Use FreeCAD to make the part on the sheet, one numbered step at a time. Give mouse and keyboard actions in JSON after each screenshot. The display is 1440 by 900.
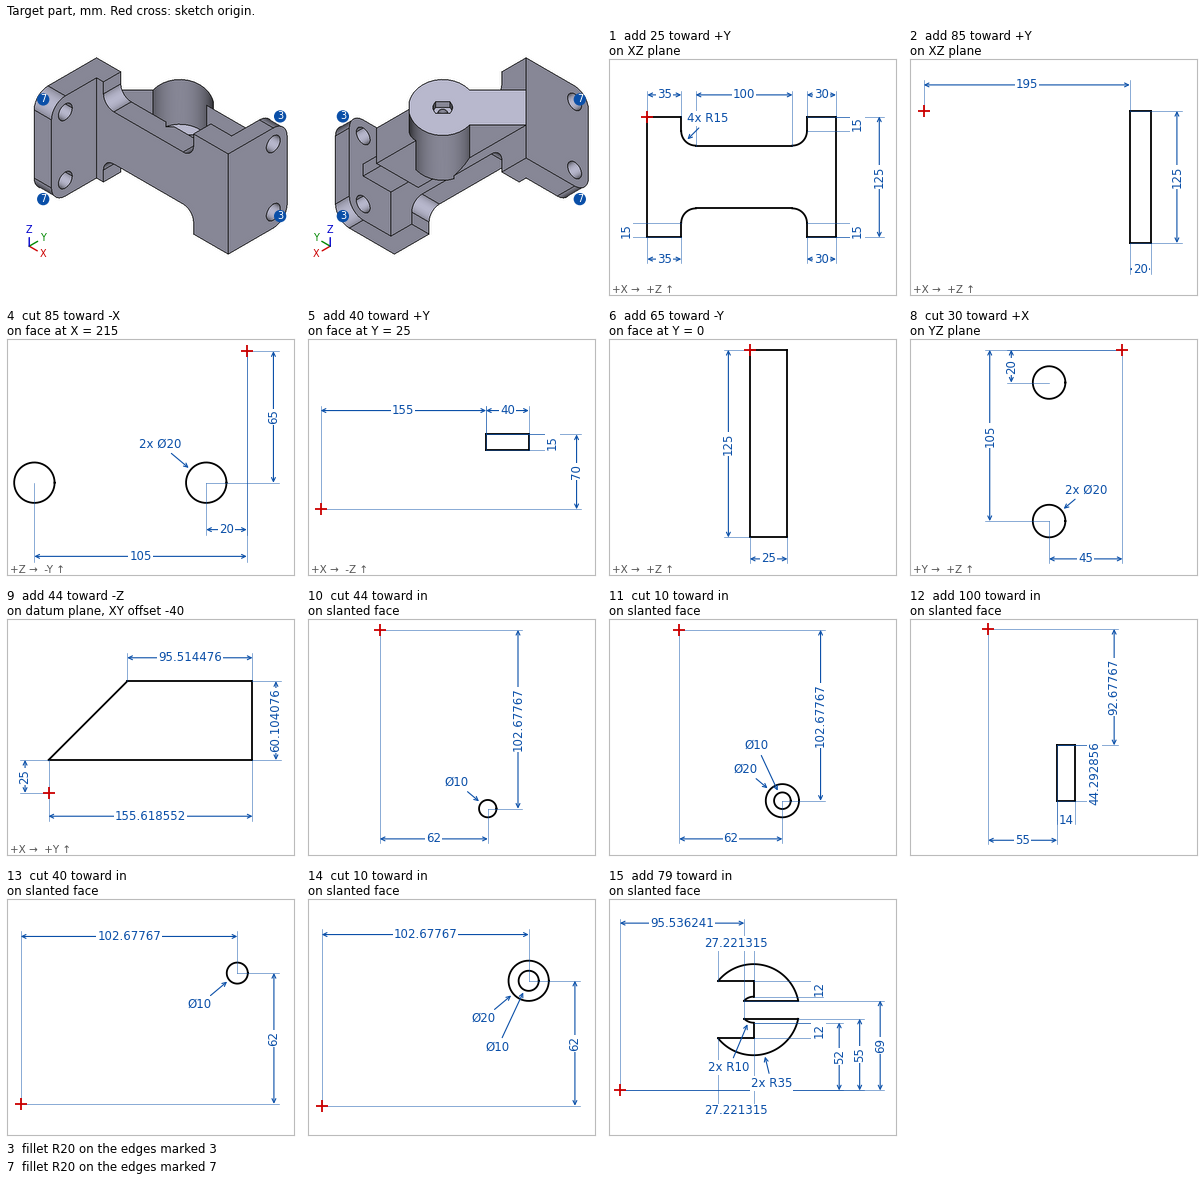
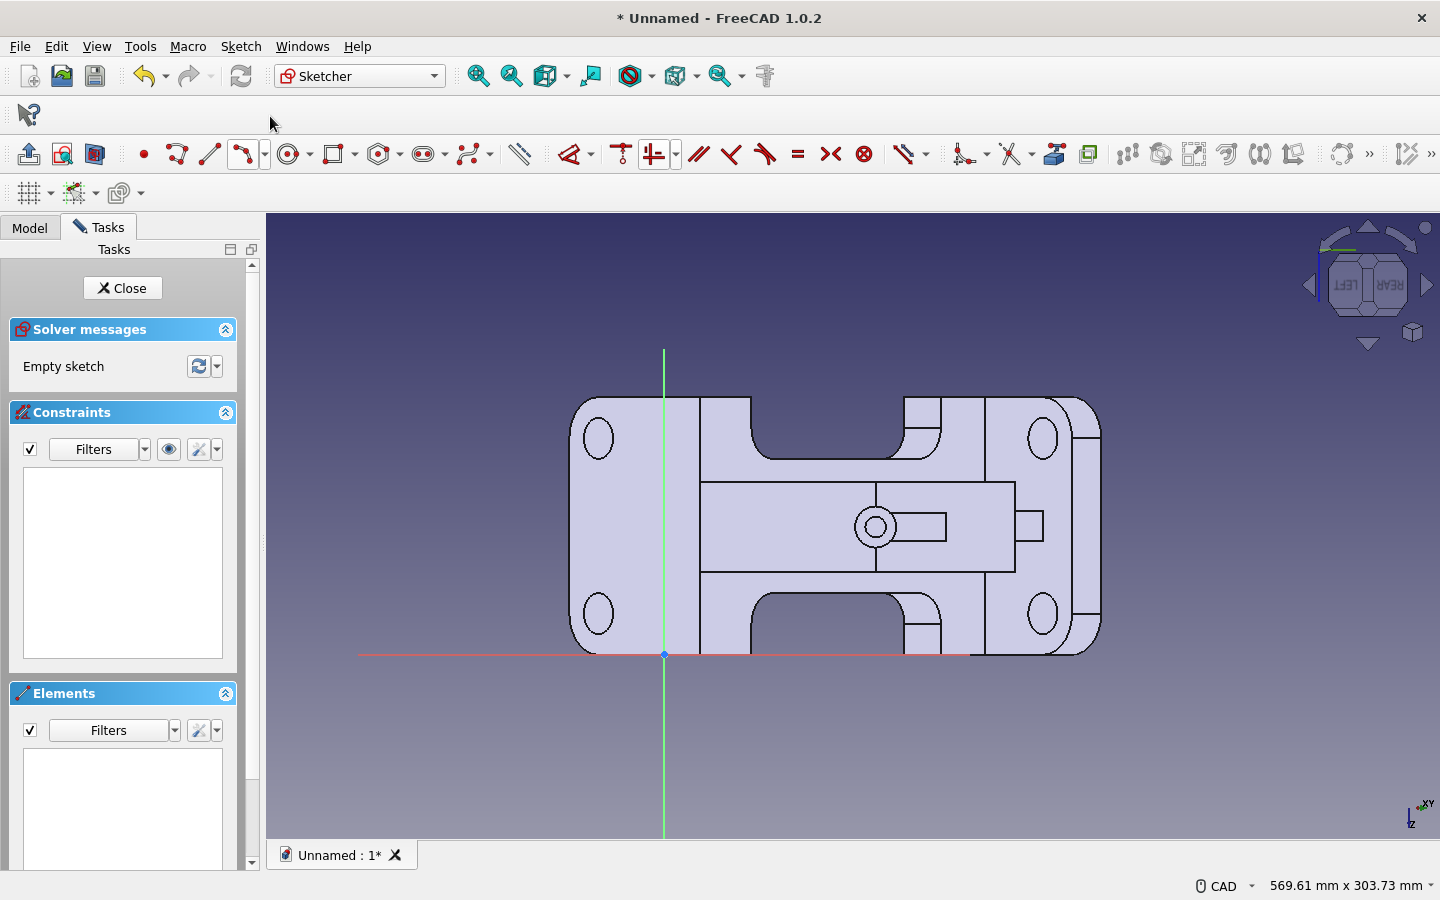
{"action": "scroll", "coordinate": [822, 580], "scroll_direction": "up", "scroll_amount": 4}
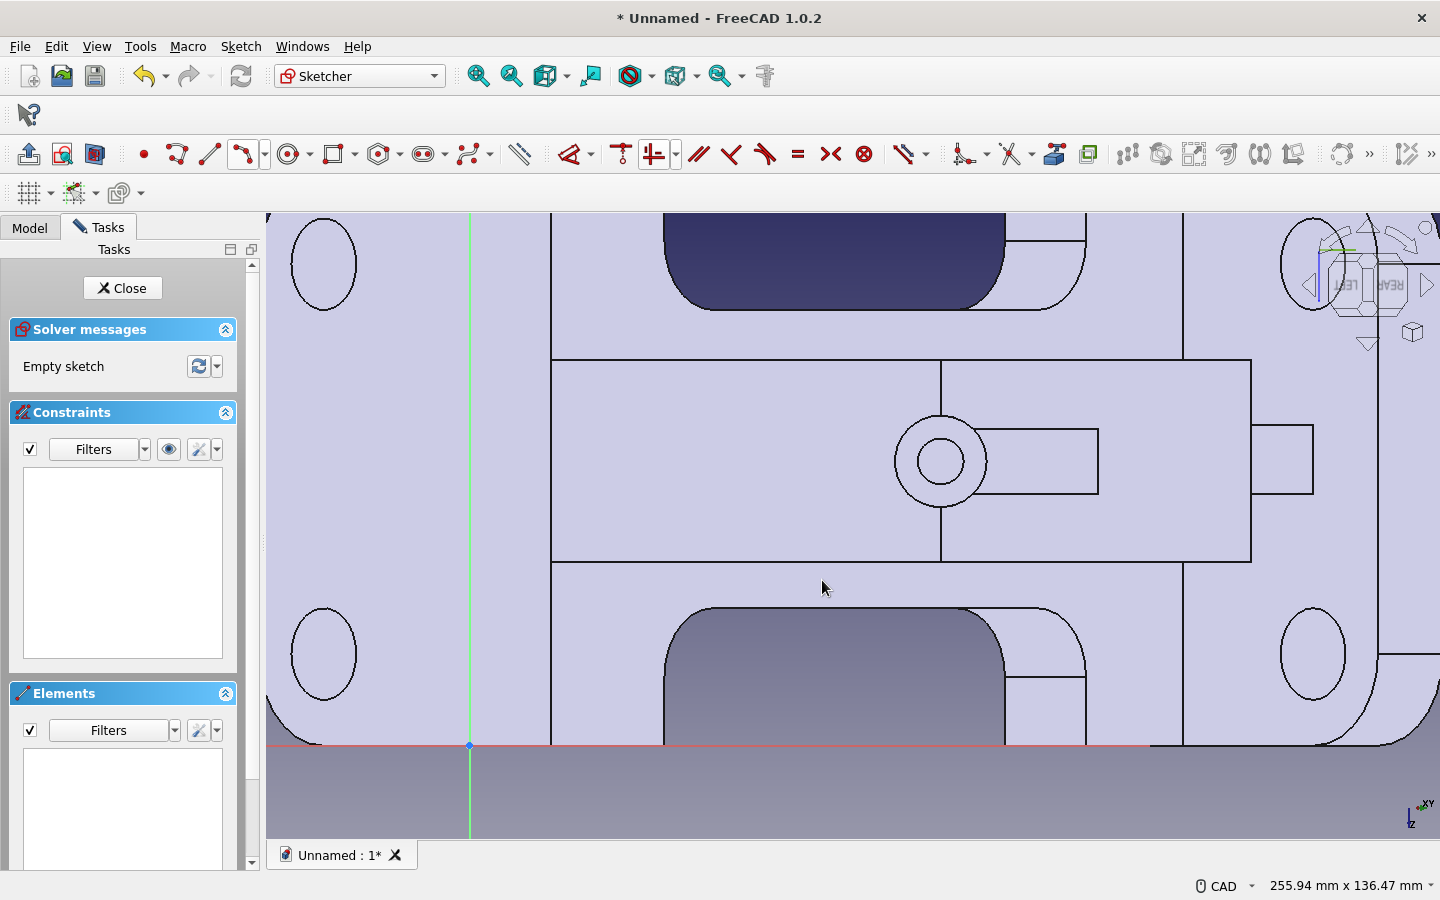
{"action": "left_click", "coordinate": [210, 154]}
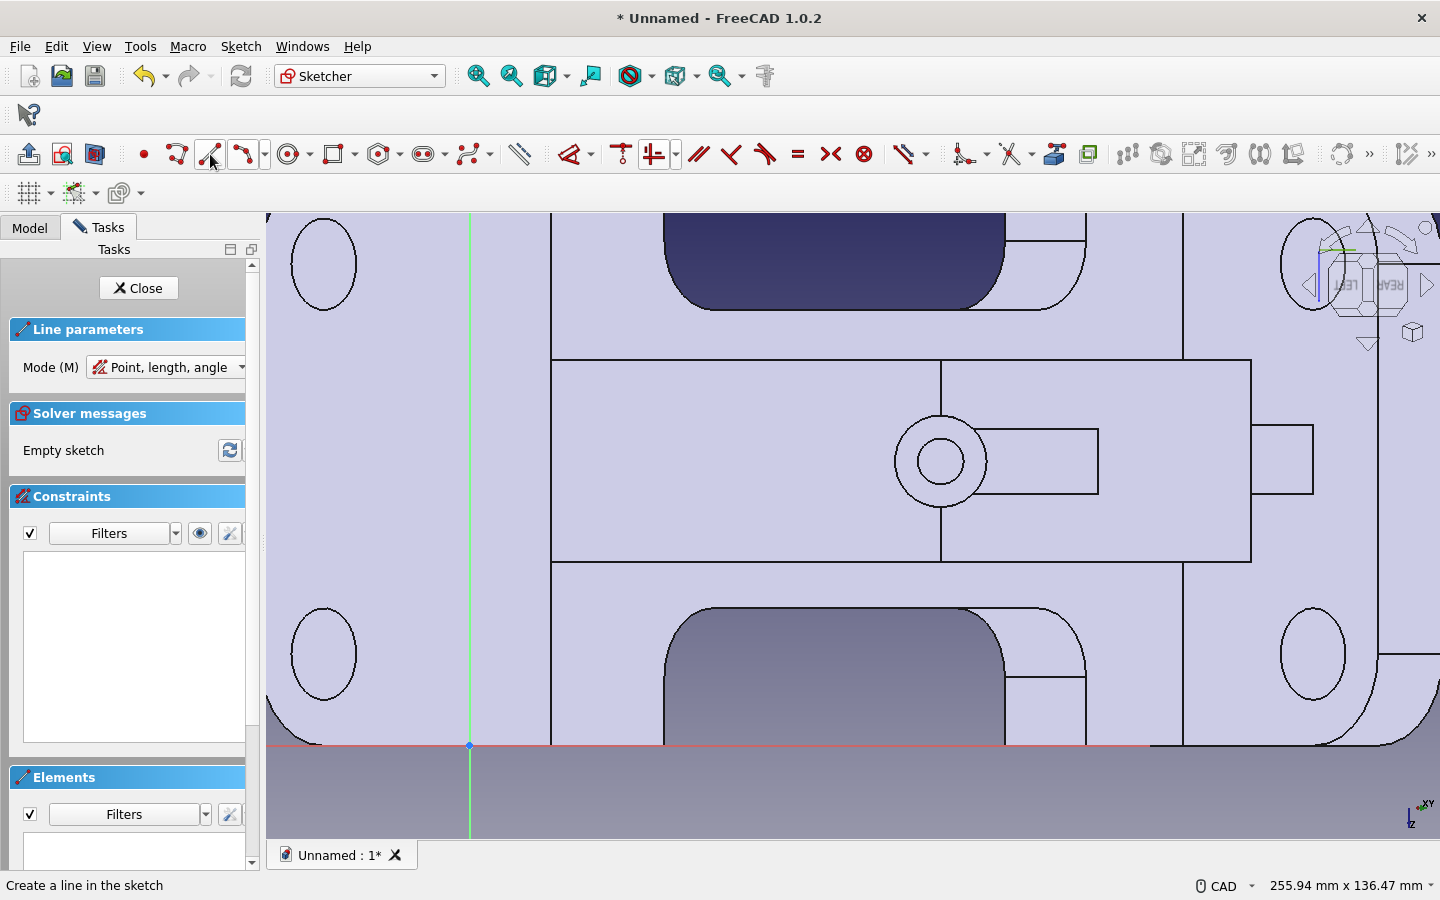
{"action": "left_click", "coordinate": [1098, 494]}
{"action": "left_click", "coordinate": [908, 494]}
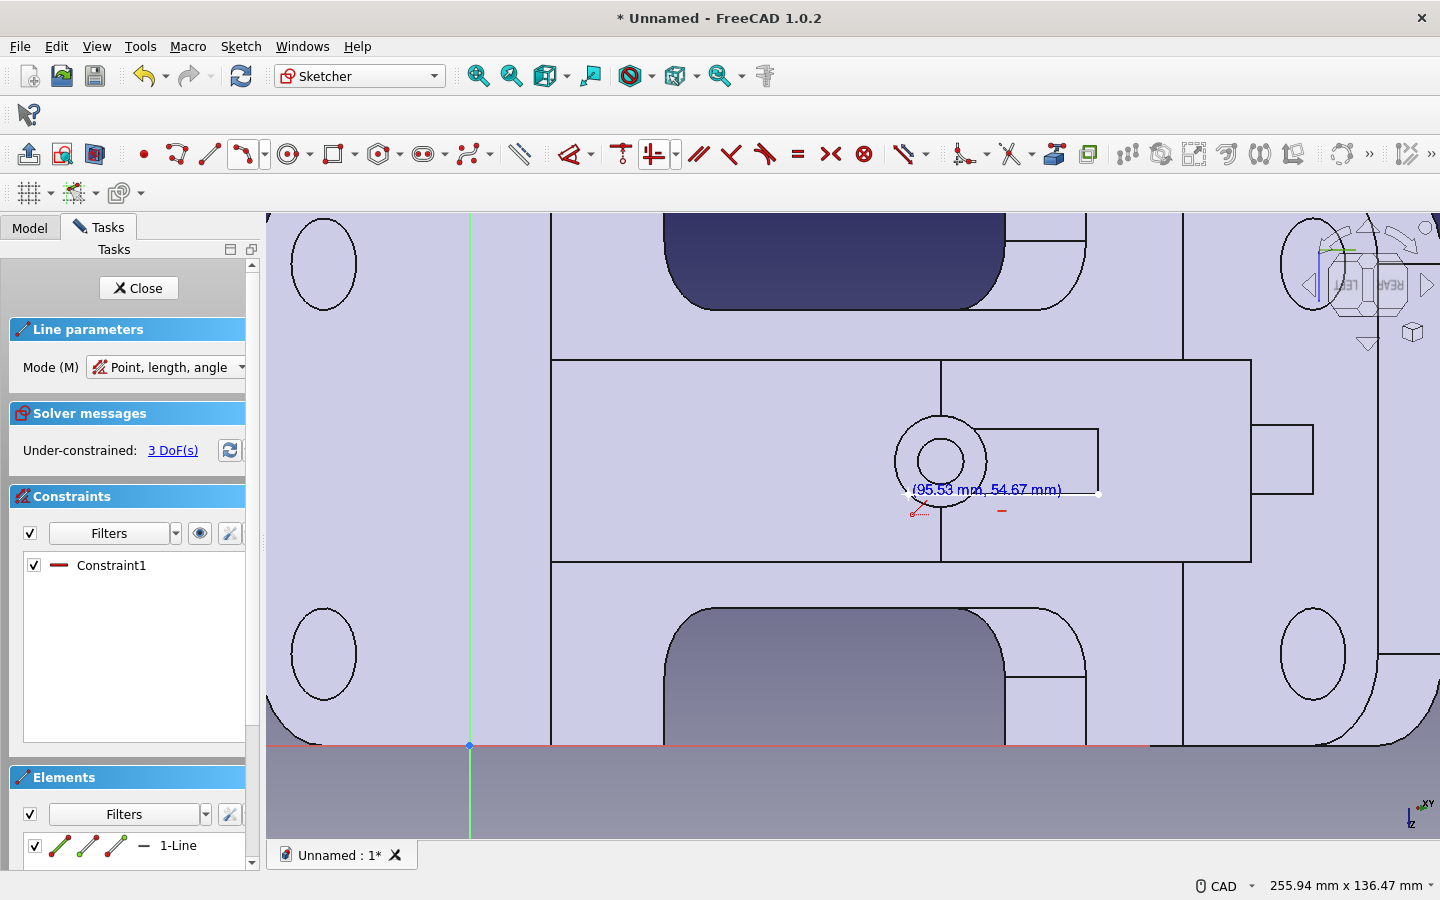
{"action": "left_click", "coordinate": [177, 154]}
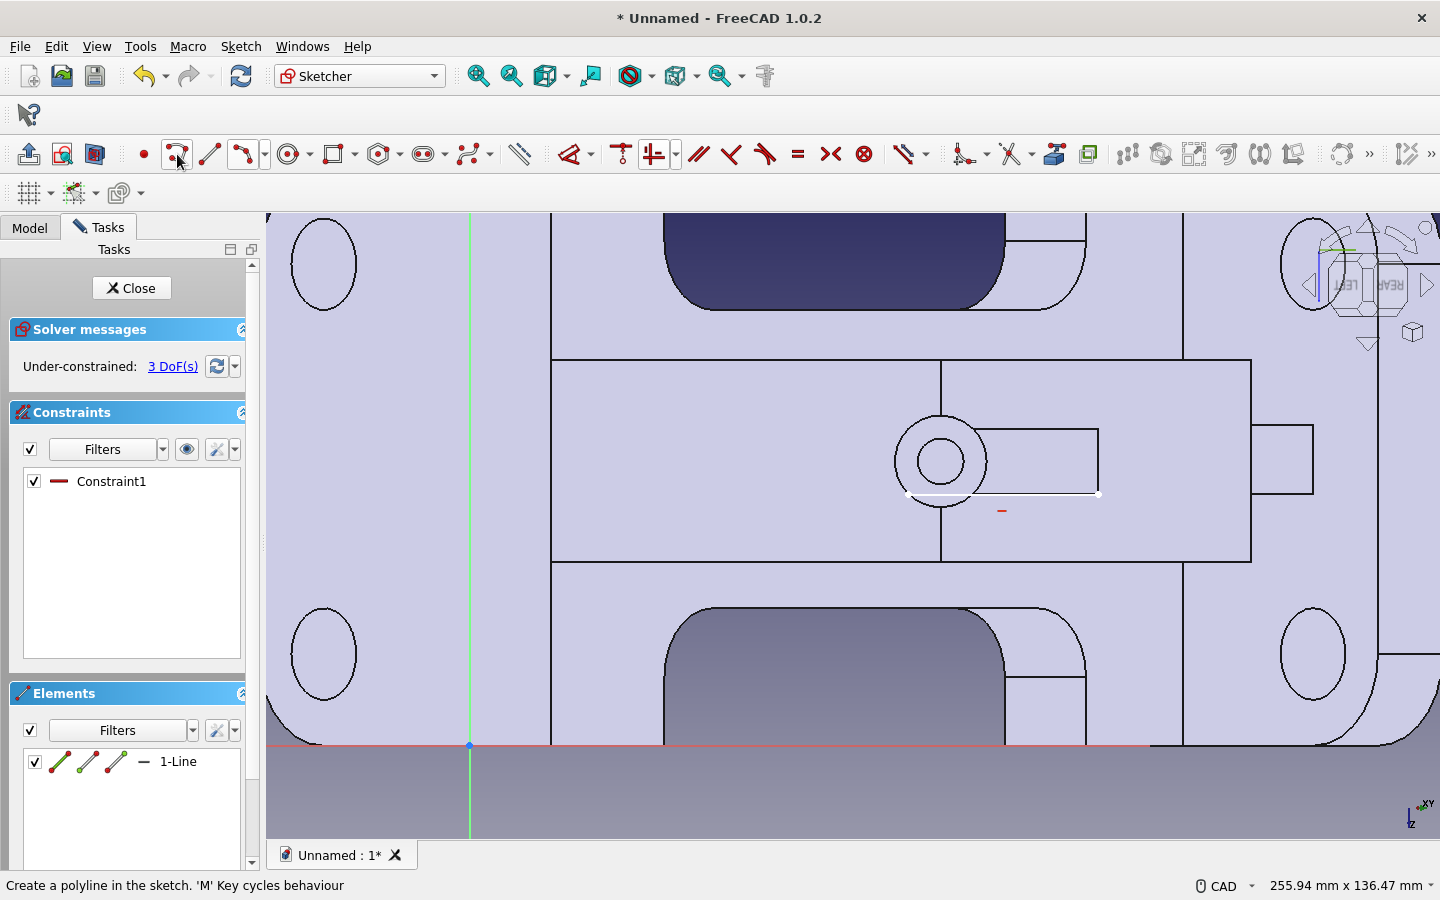
{"action": "left_click", "coordinate": [941, 507]}
{"action": "left_click", "coordinate": [941, 562]}
{"action": "left_click", "coordinate": [816, 562]}
{"action": "right_click", "coordinate": [816, 562]}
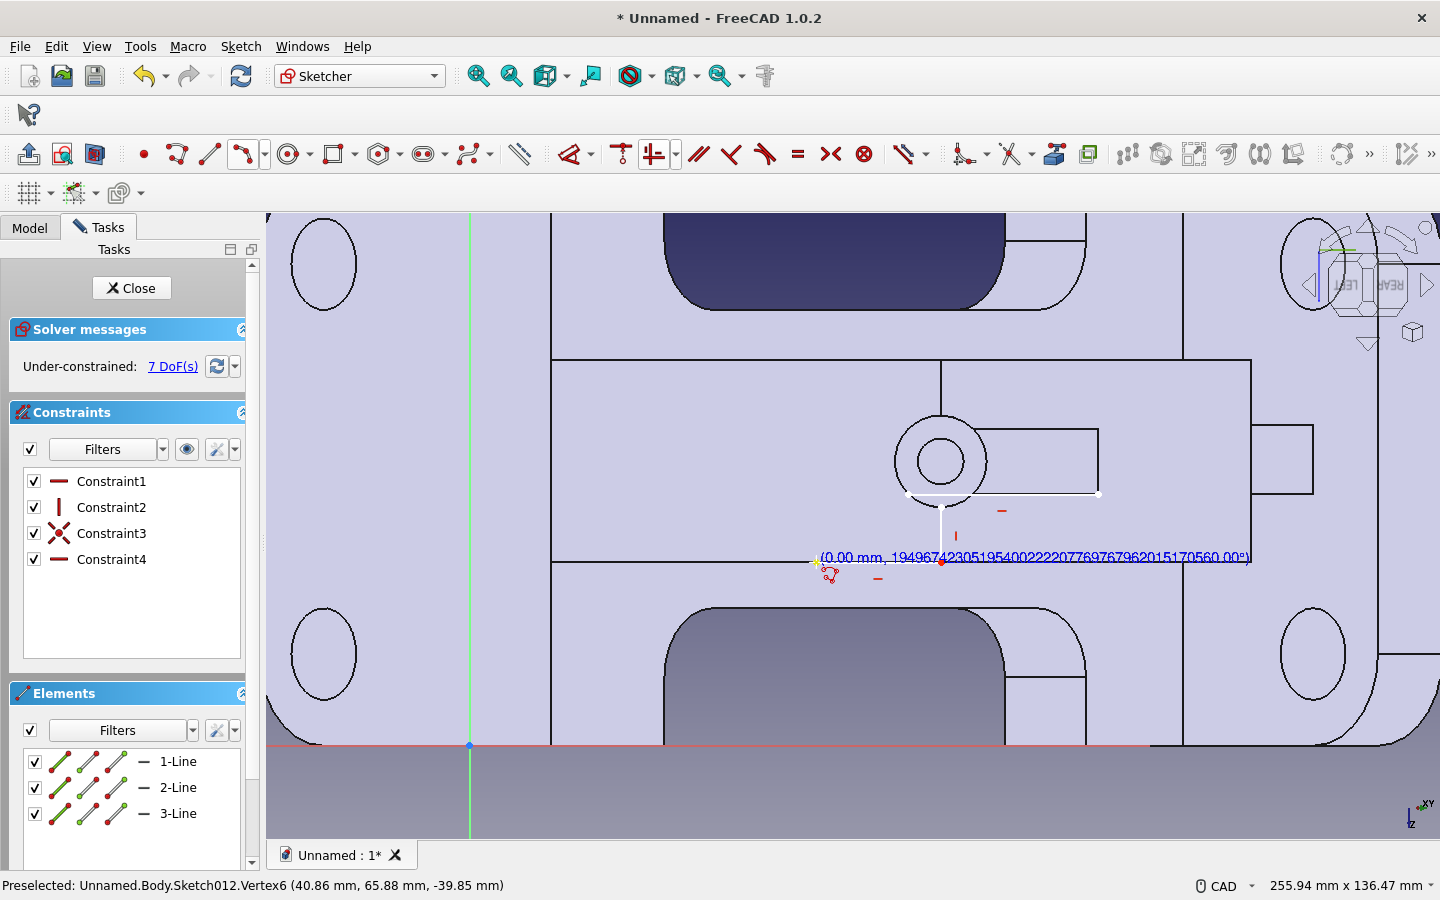
{"action": "left_click", "coordinate": [242, 154]}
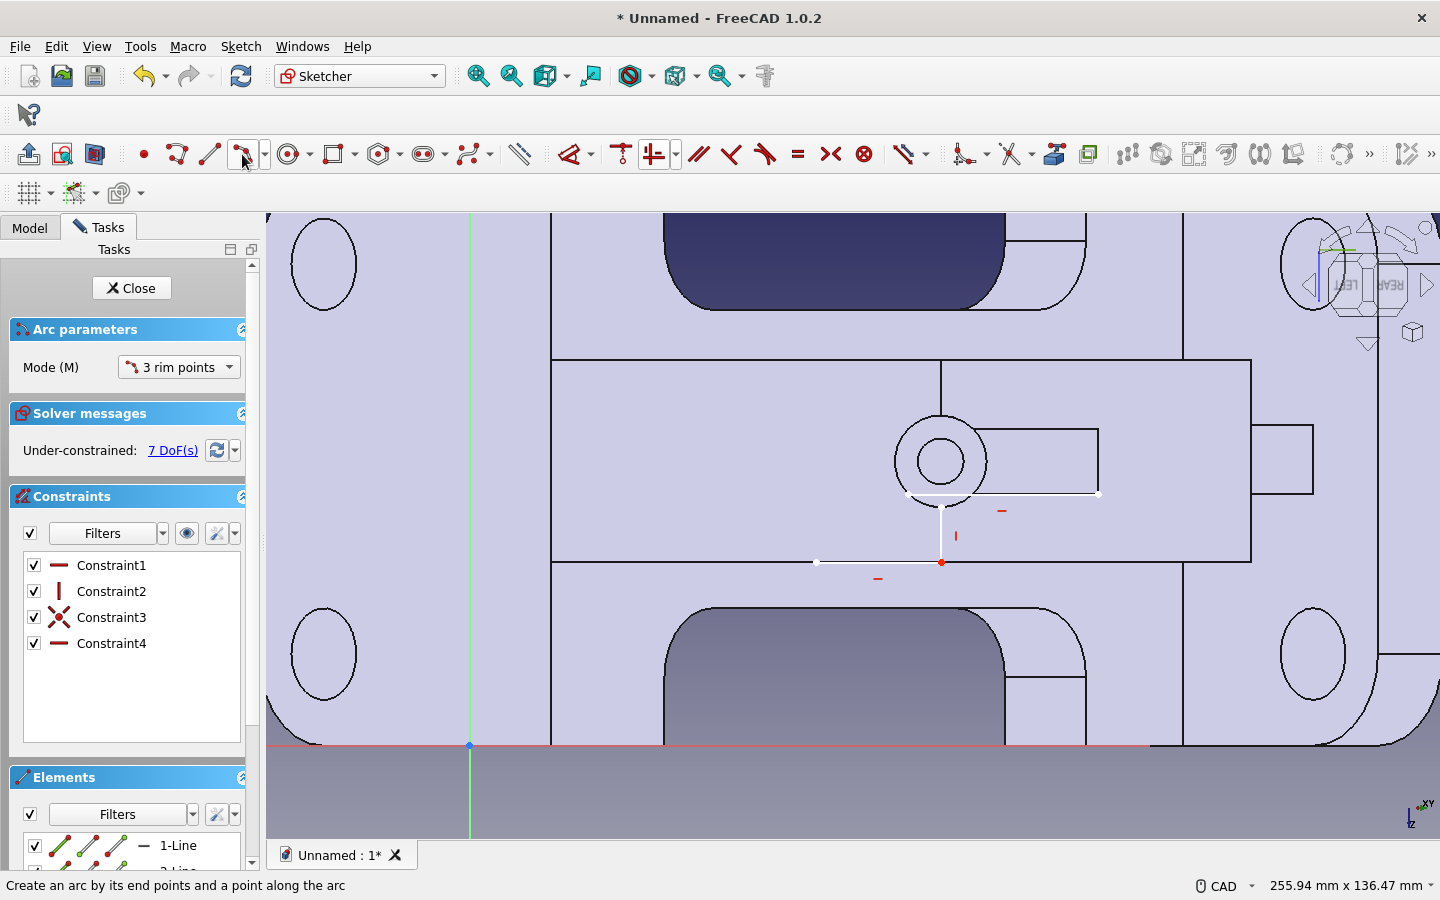
{"action": "left_click", "coordinate": [908, 495]}
{"action": "left_click", "coordinate": [941, 508]}